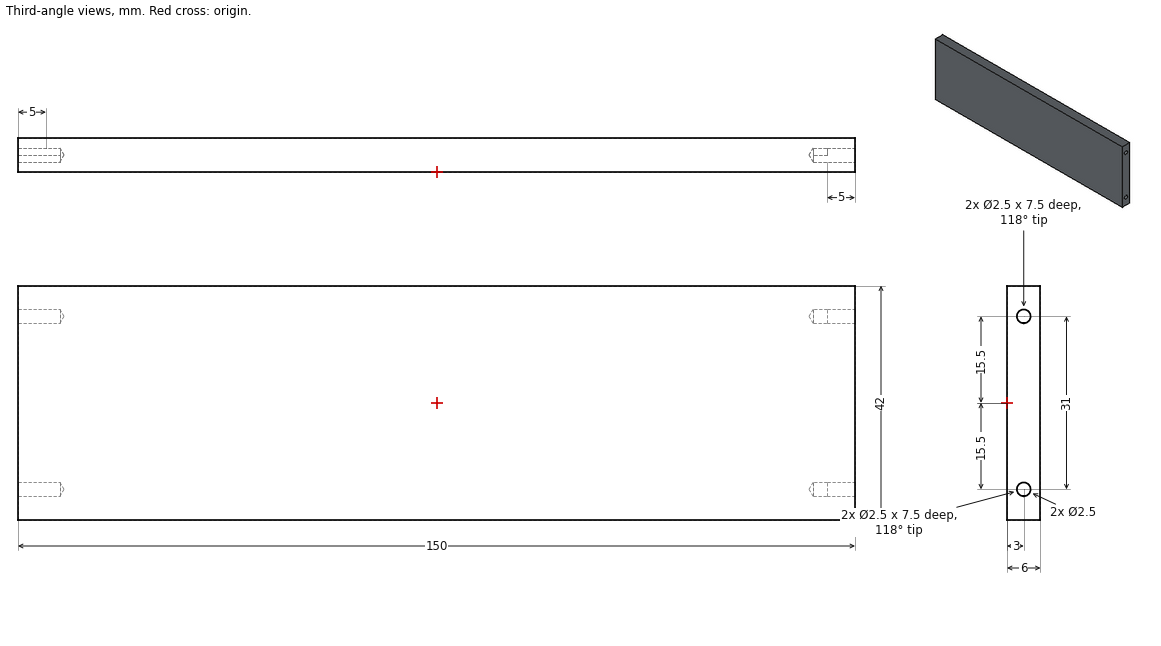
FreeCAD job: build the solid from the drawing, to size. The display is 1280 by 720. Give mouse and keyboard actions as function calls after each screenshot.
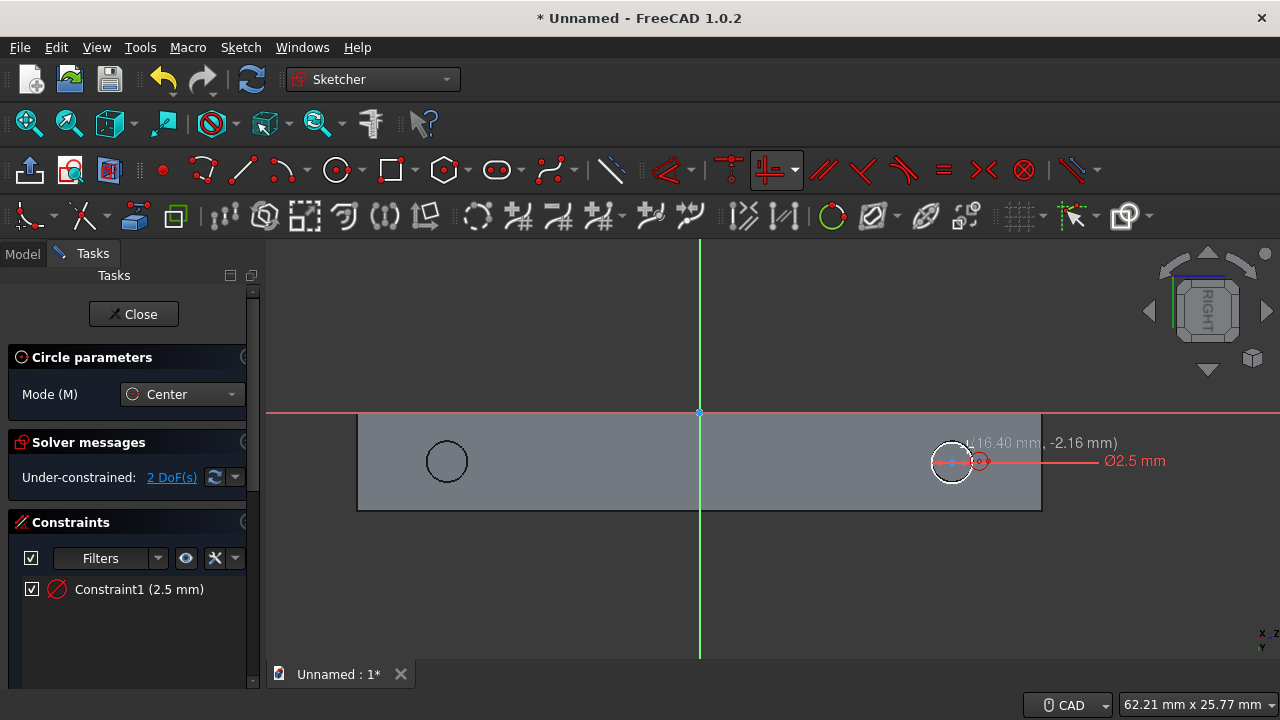
click(447, 462)
move(461, 447)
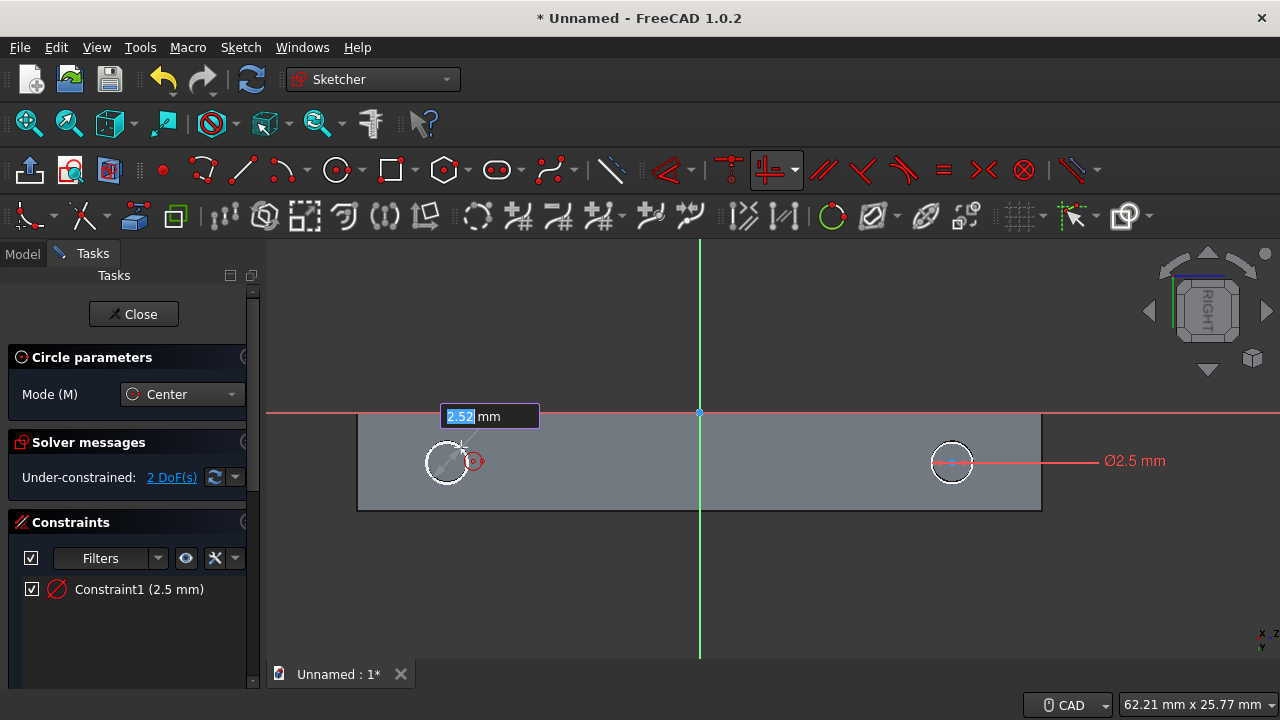
text(2.5)
key(Return)
key(Escape)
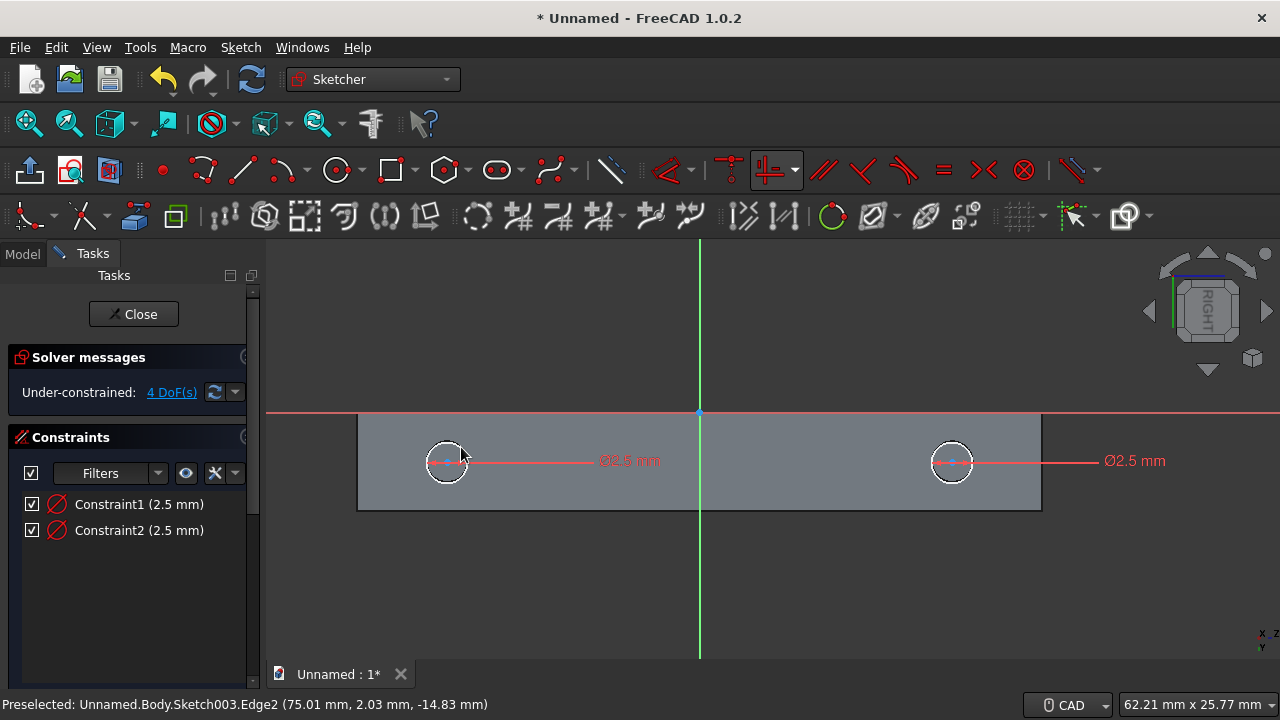
click(952, 463)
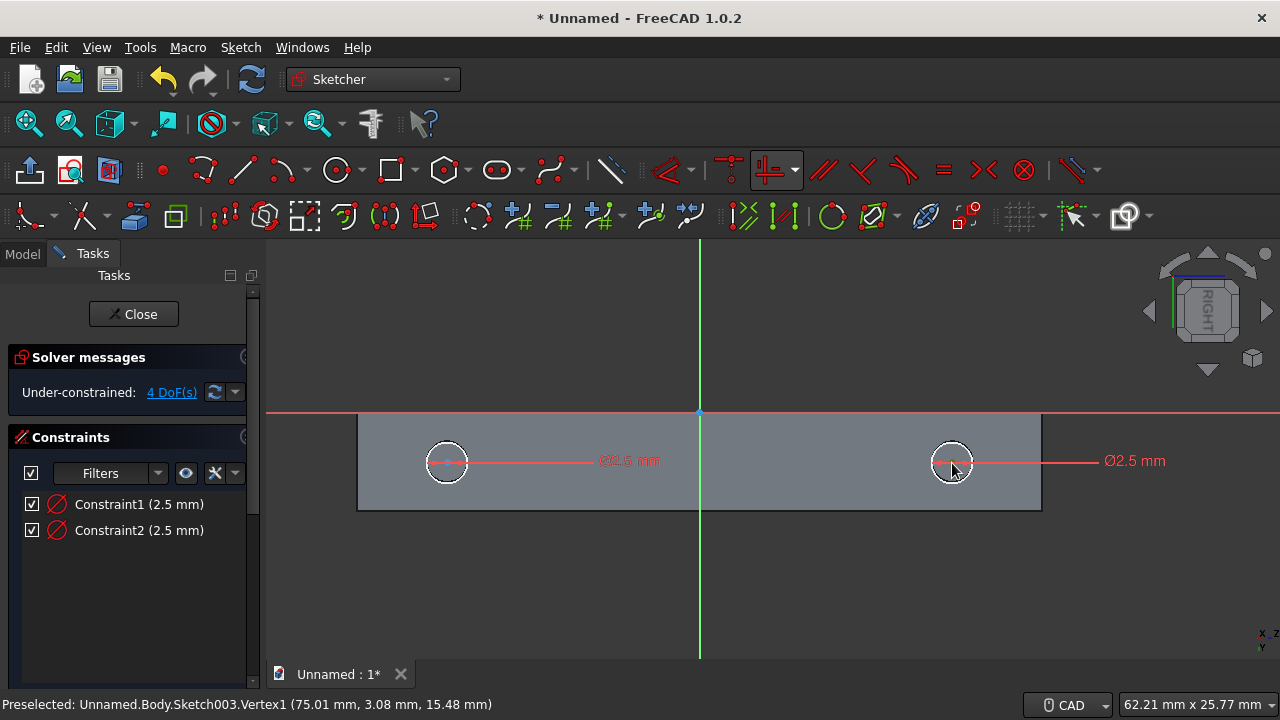
click(447, 463)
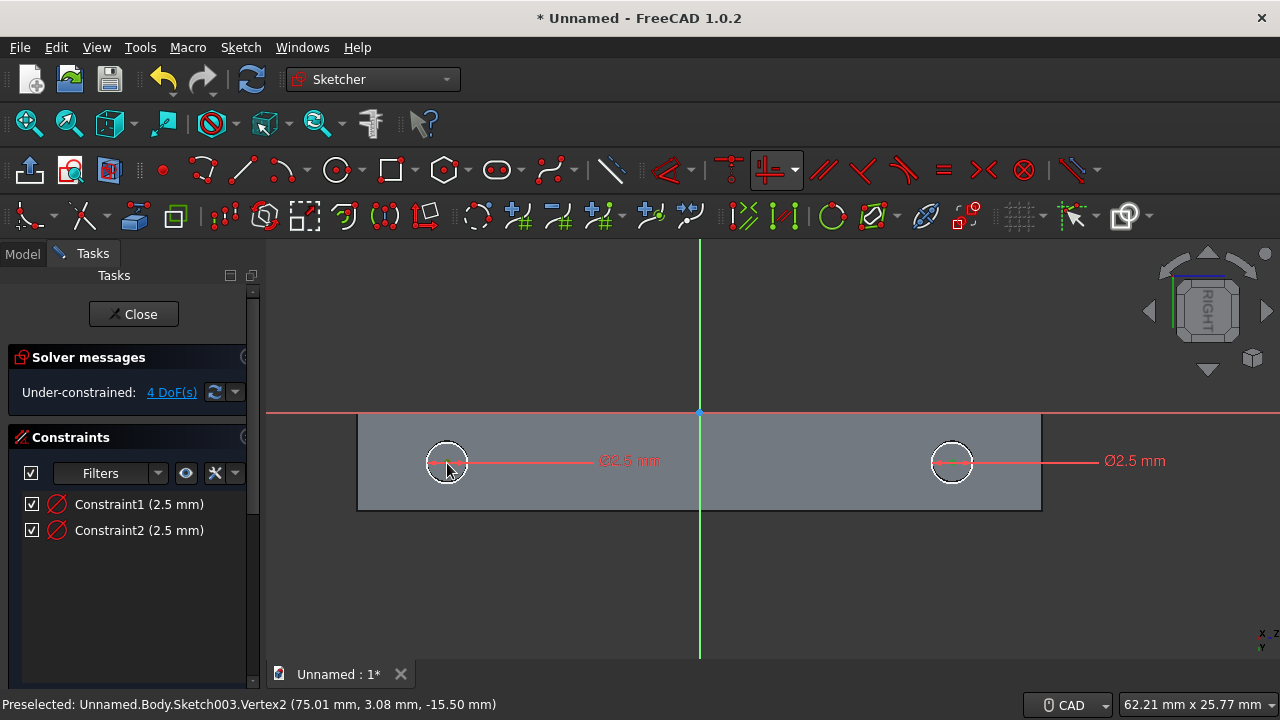
click(798, 170)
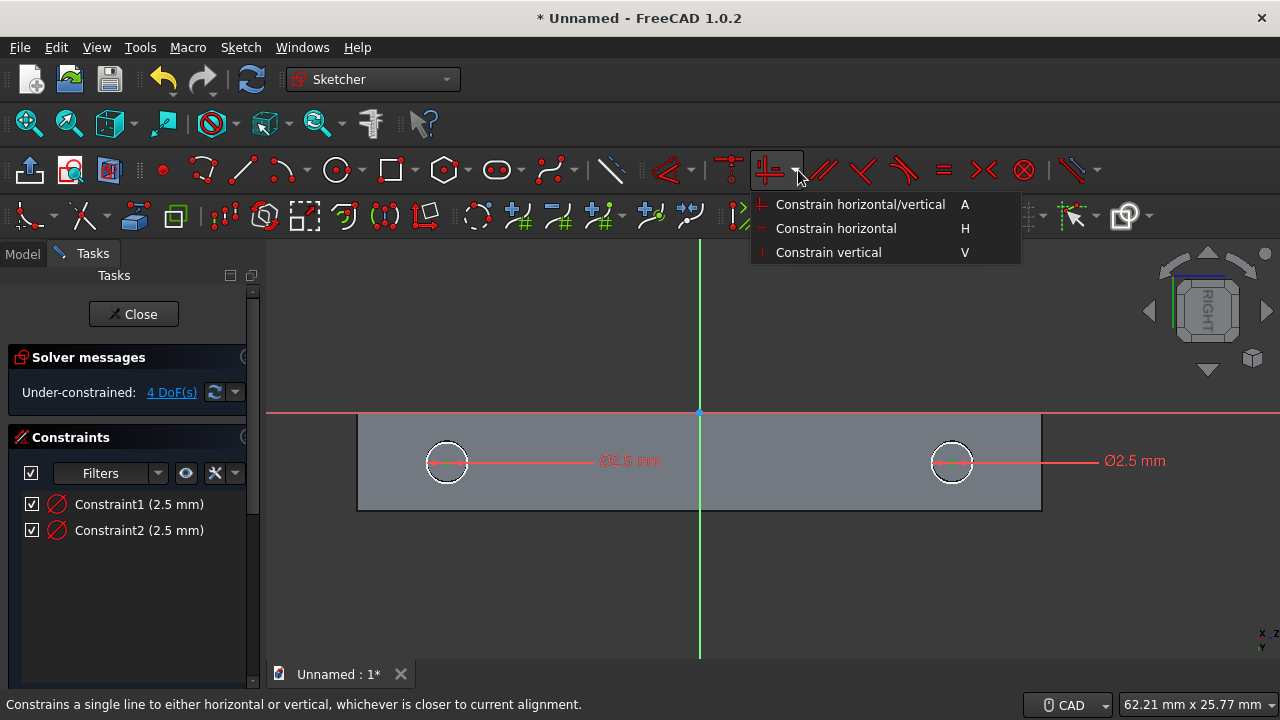
click(886, 228)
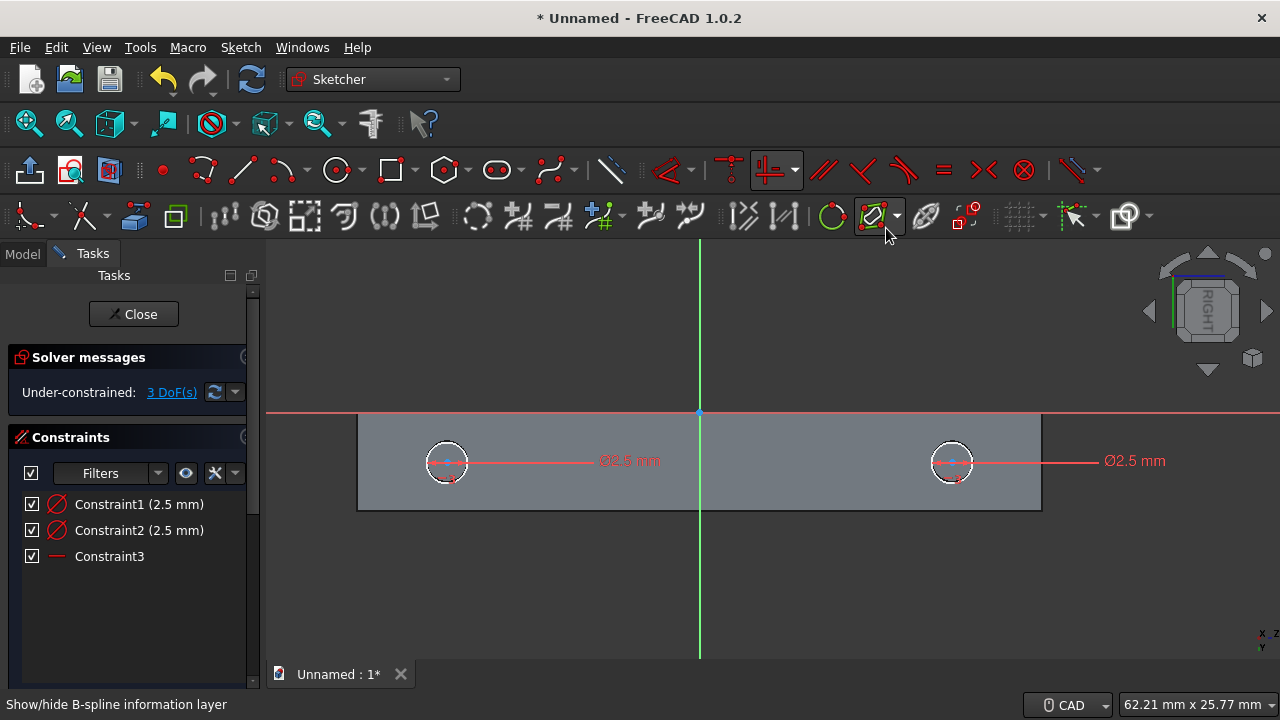
click(666, 170)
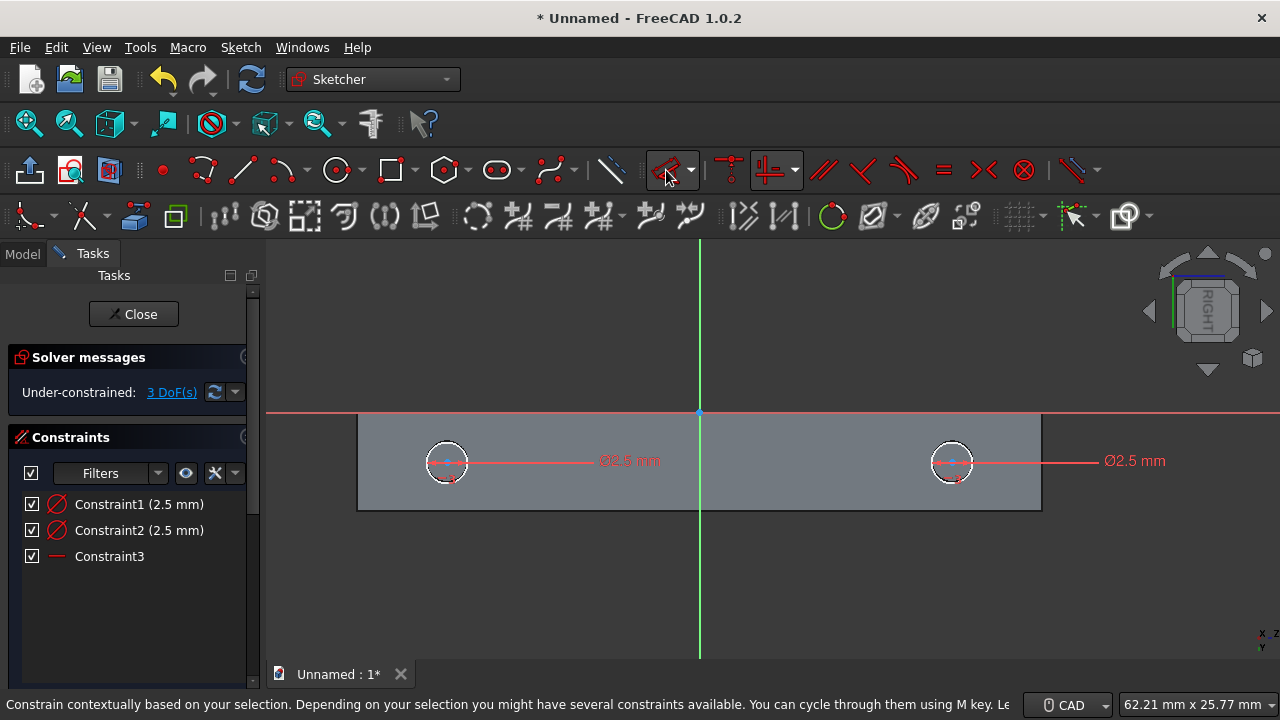
click(952, 463)
click(986, 438)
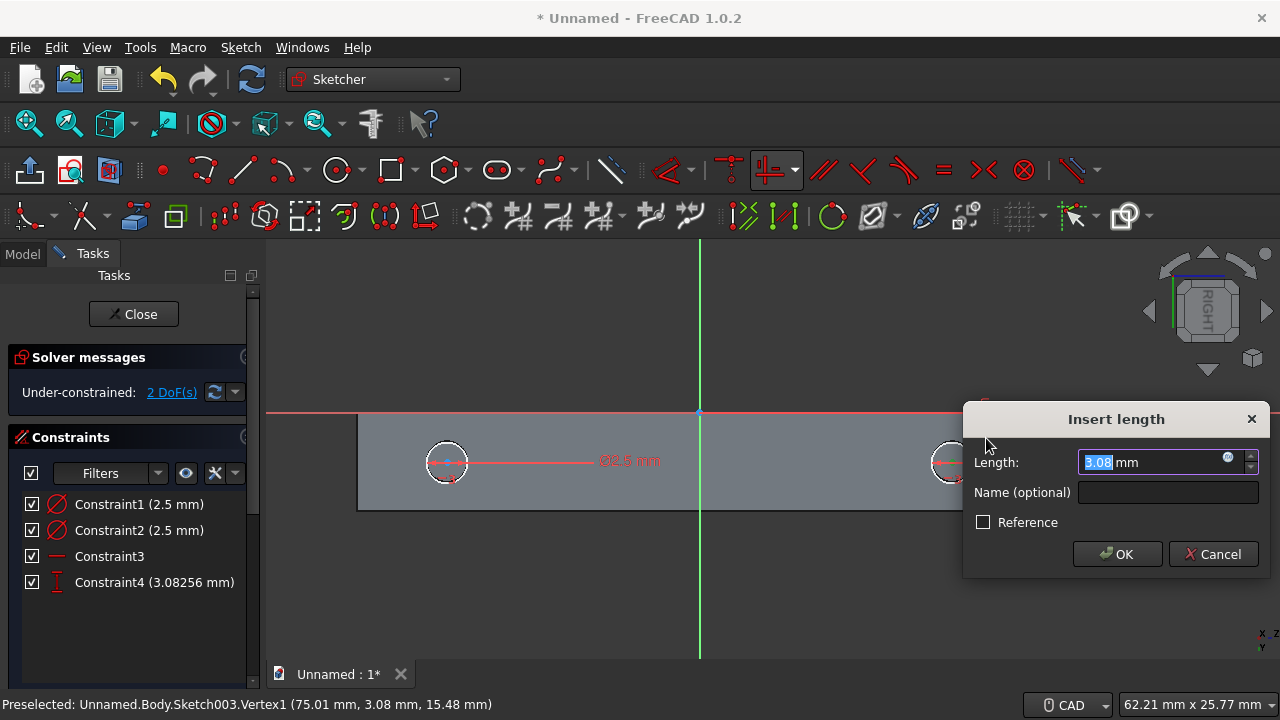
text(3)
key(Return)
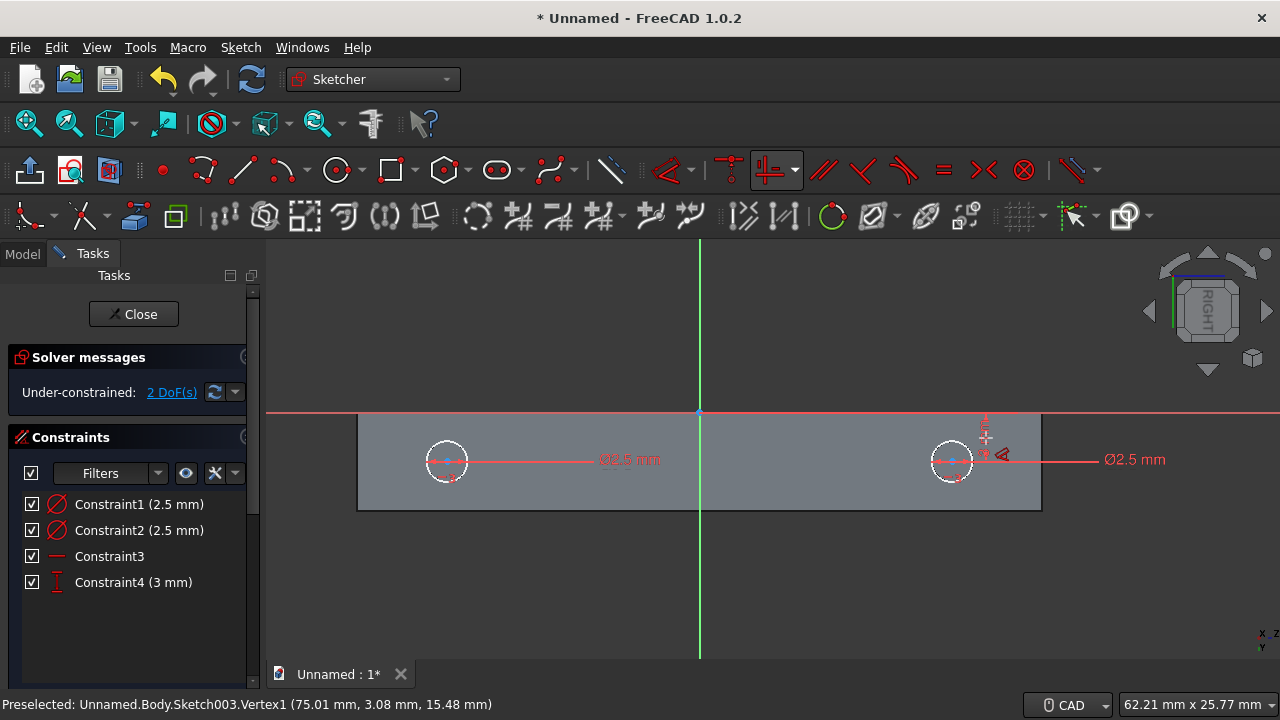
click(952, 462)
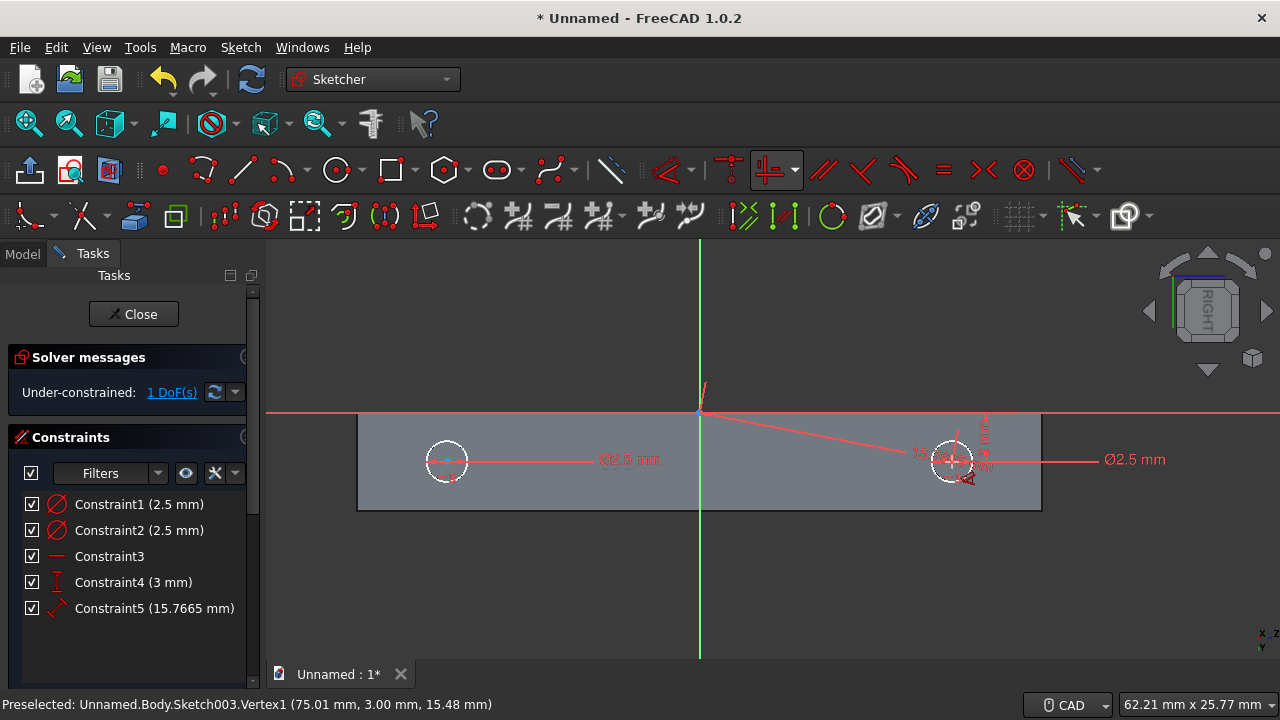
click(447, 462)
click(583, 496)